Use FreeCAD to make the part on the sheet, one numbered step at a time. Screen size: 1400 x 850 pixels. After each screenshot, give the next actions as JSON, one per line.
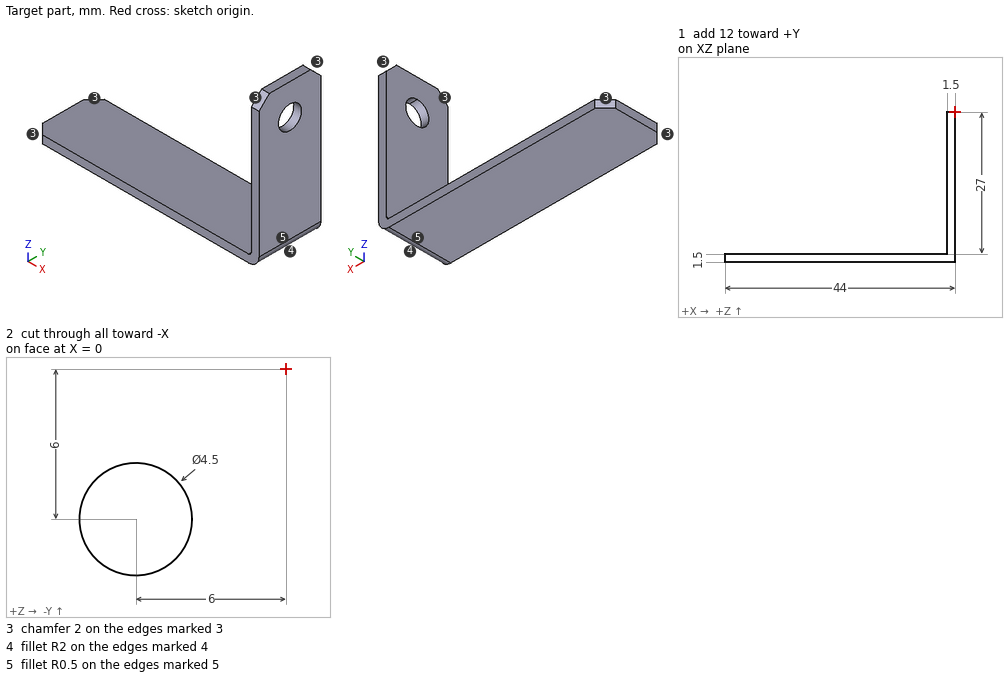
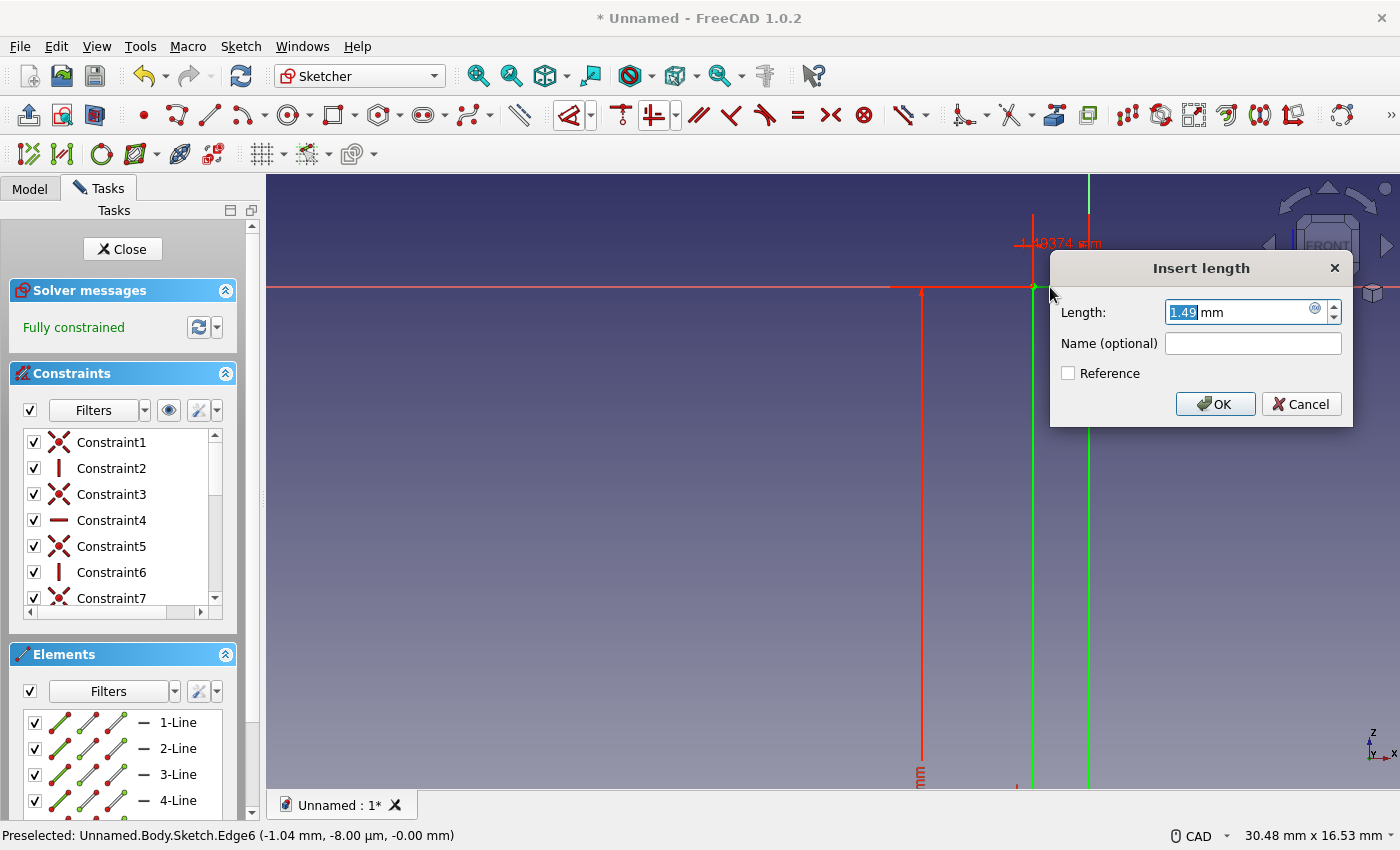
{"action": "type", "text": "1.5"}
{"action": "key", "text": "Return"}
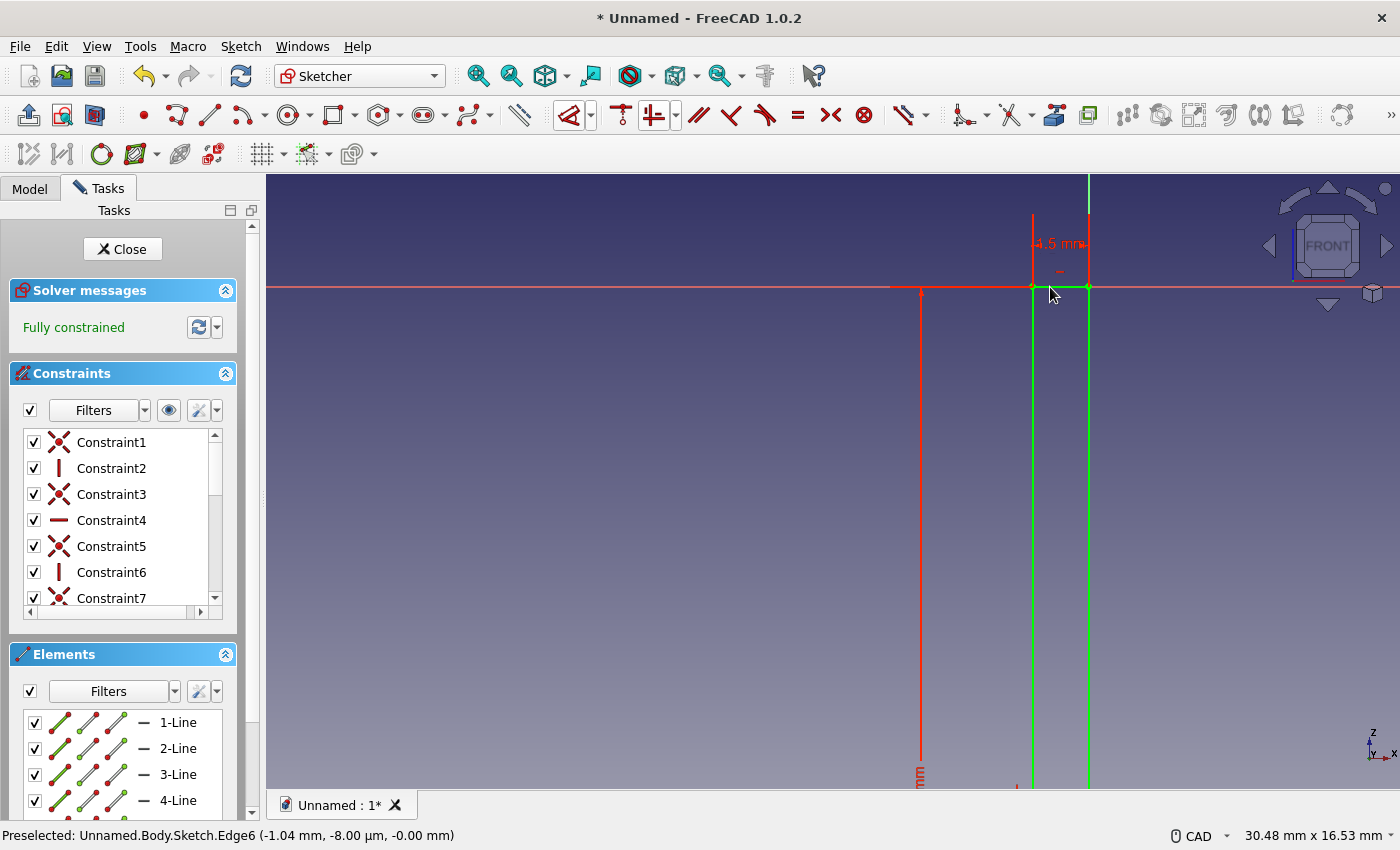
{"action": "left_click", "coordinate": [123, 249]}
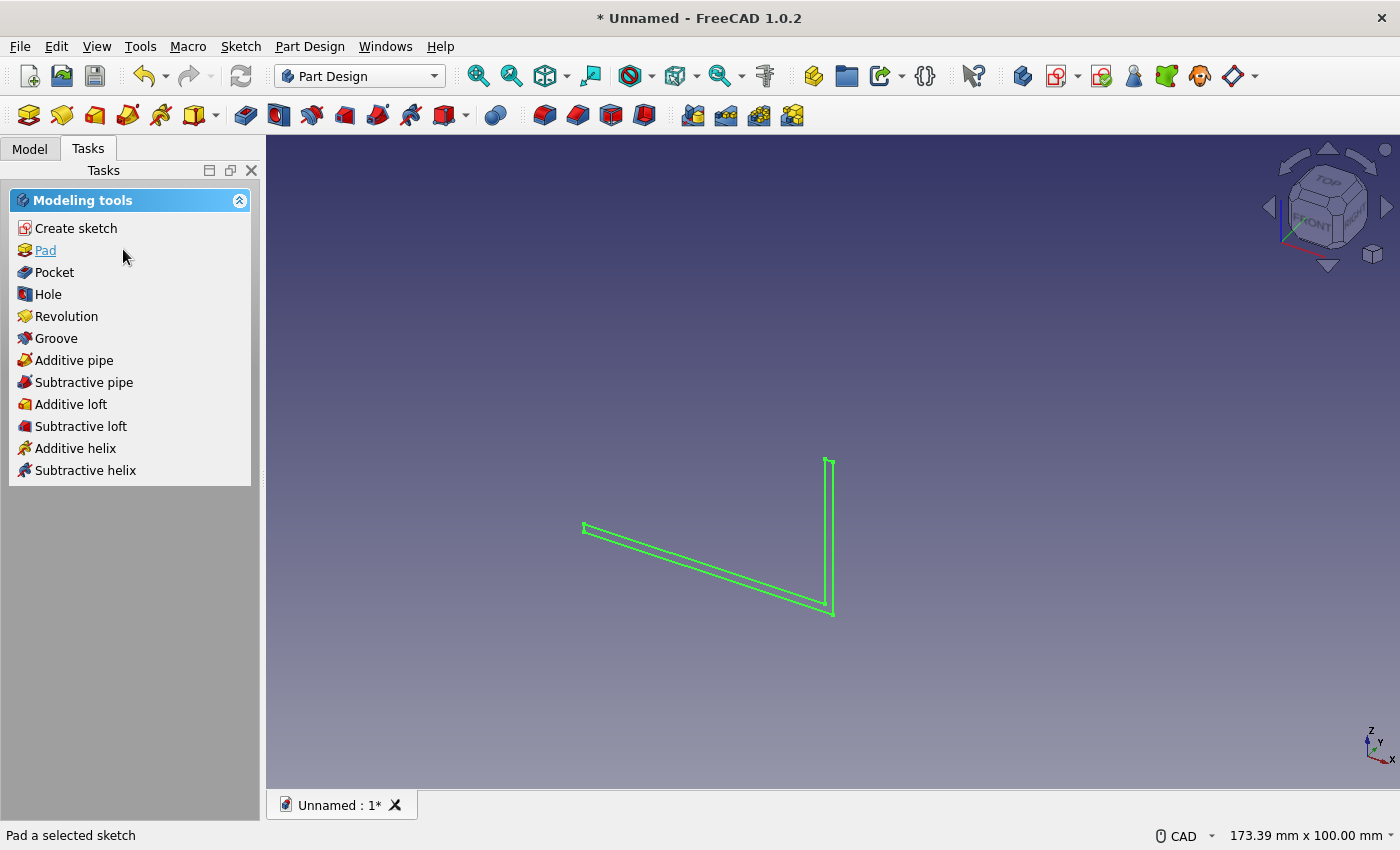
{"action": "left_click", "coordinate": [29, 116]}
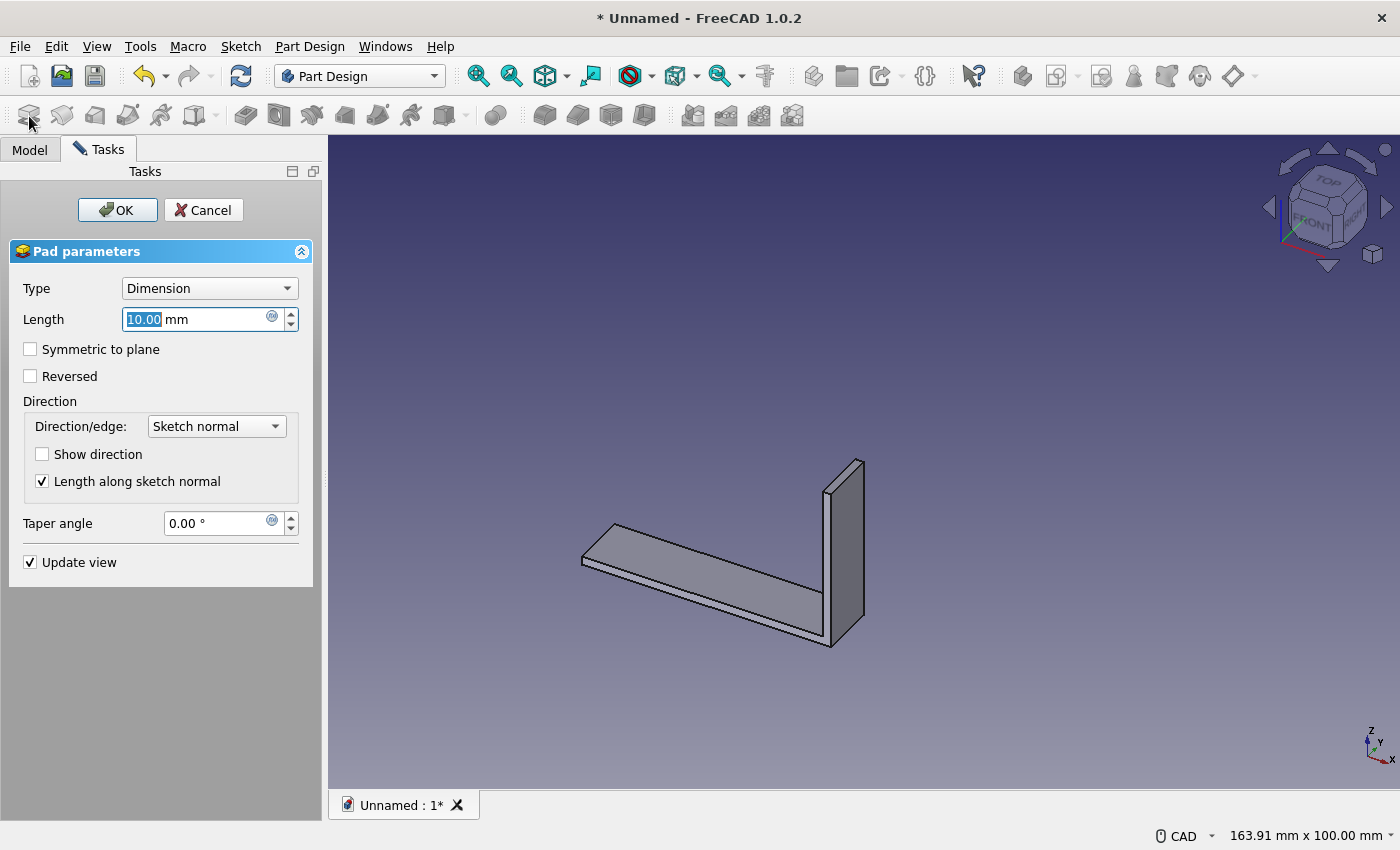
{"action": "type", "text": "12"}
{"action": "key", "text": "Tab"}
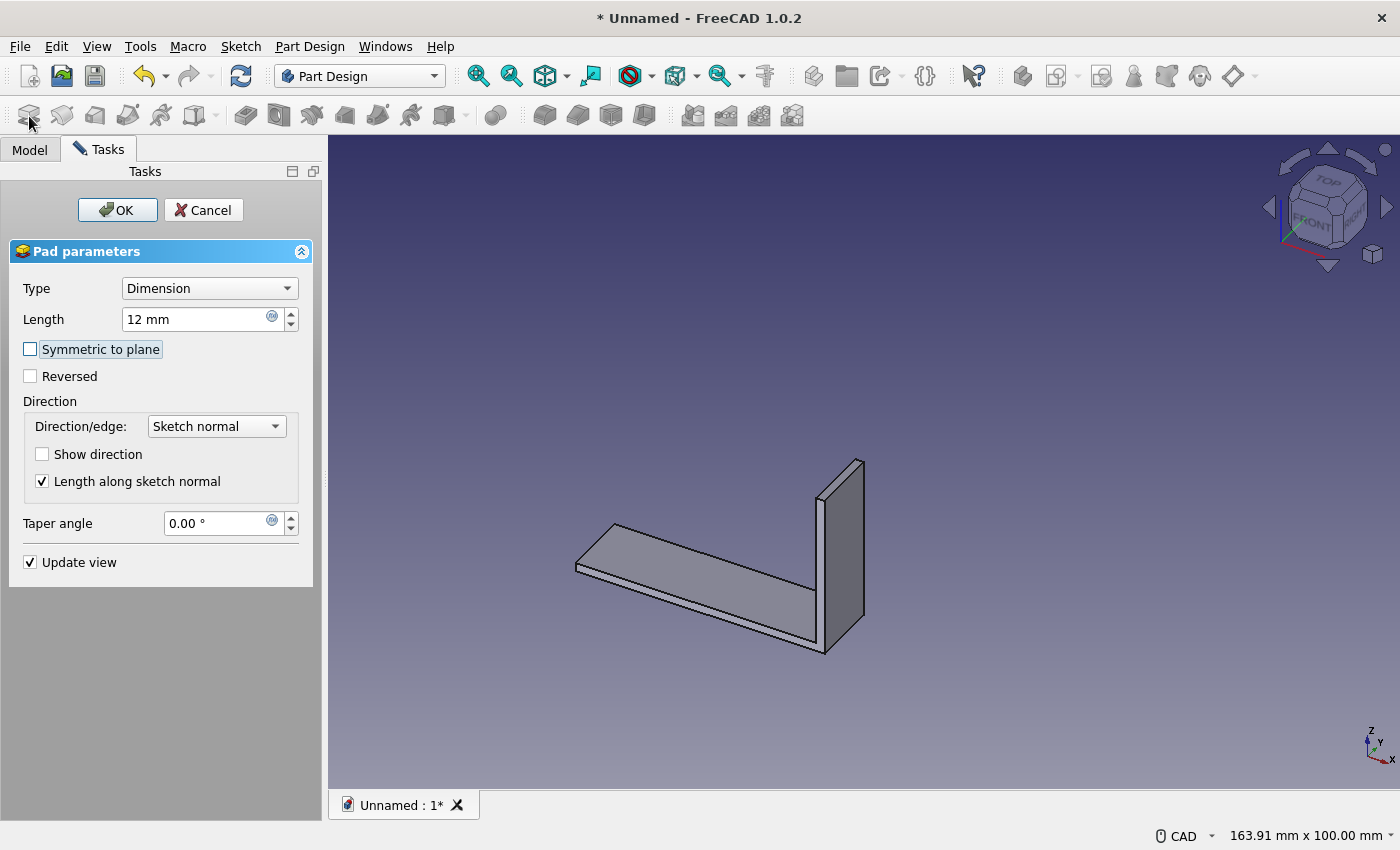
{"action": "left_click", "coordinate": [31, 376]}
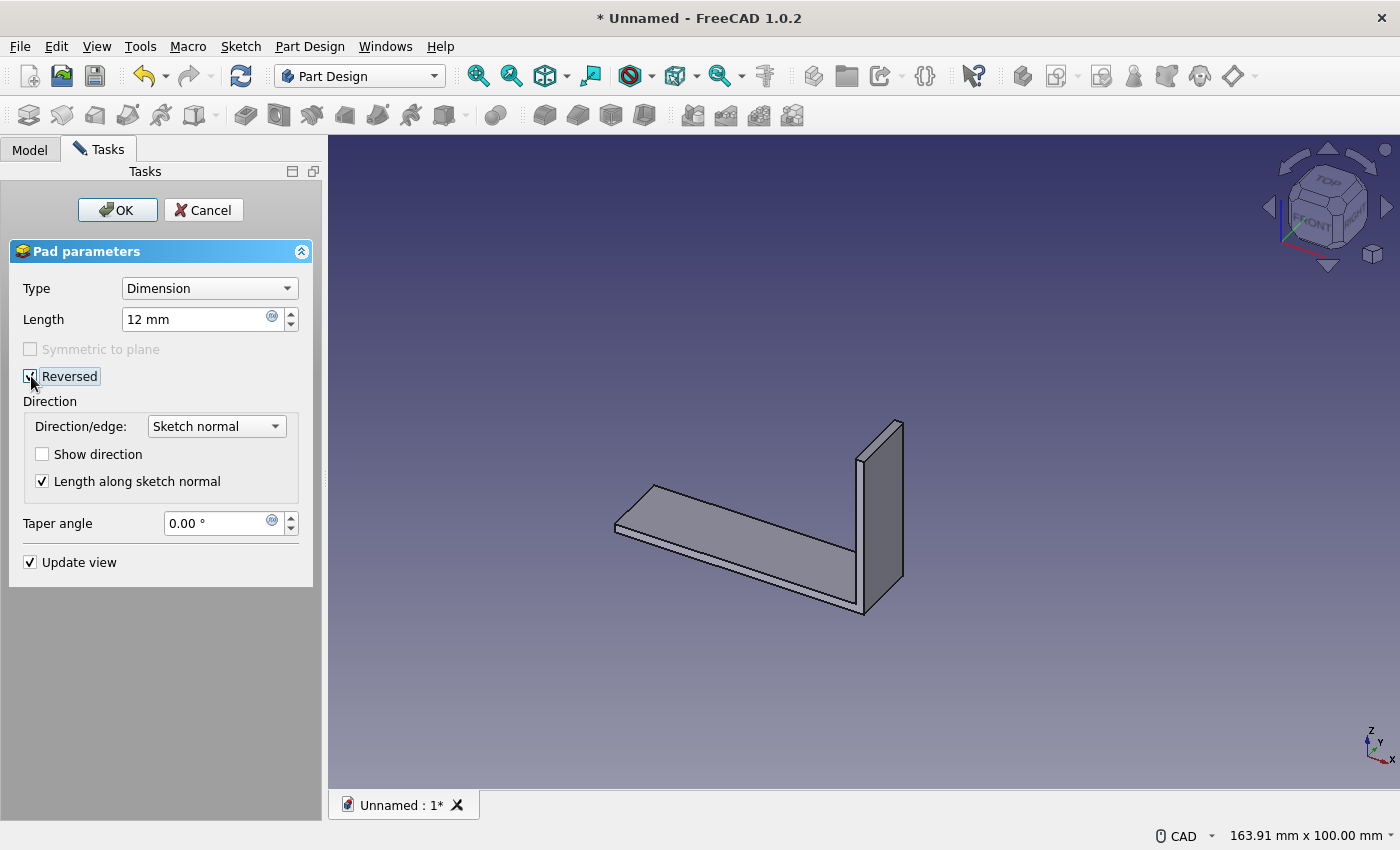
{"action": "left_click", "coordinate": [118, 210]}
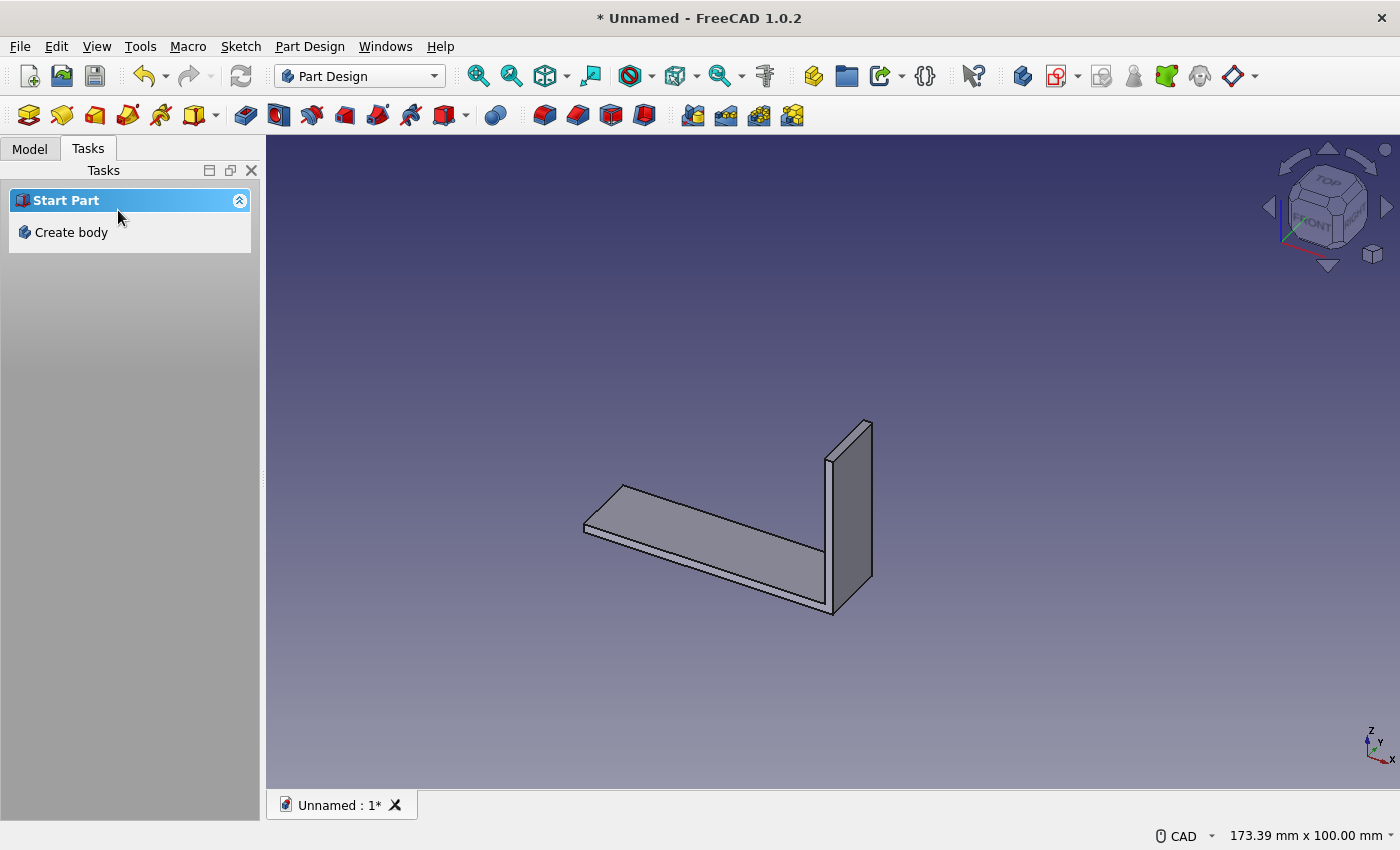
{"action": "left_click", "coordinate": [479, 76]}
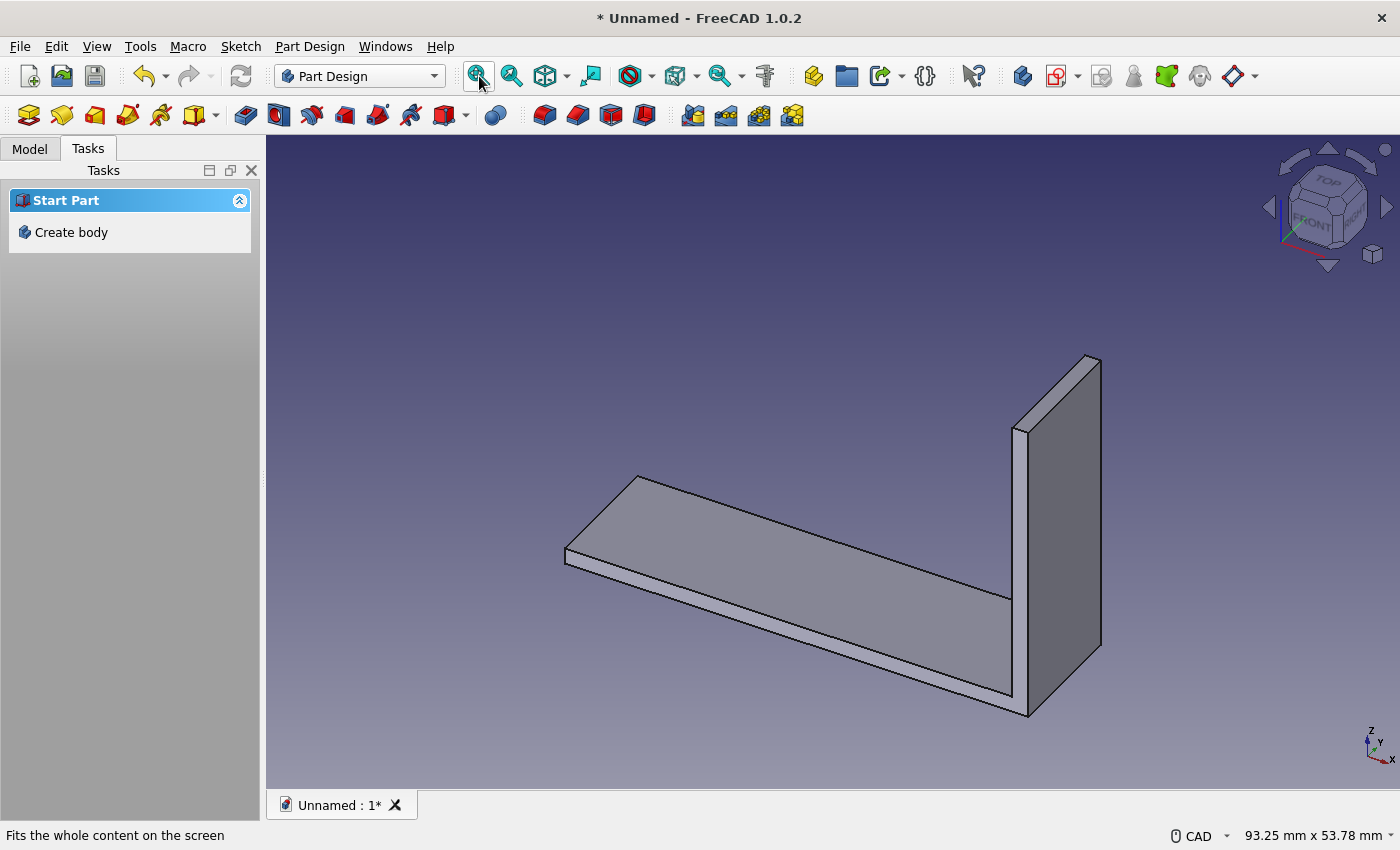
{"action": "left_click", "coordinate": [1065, 457]}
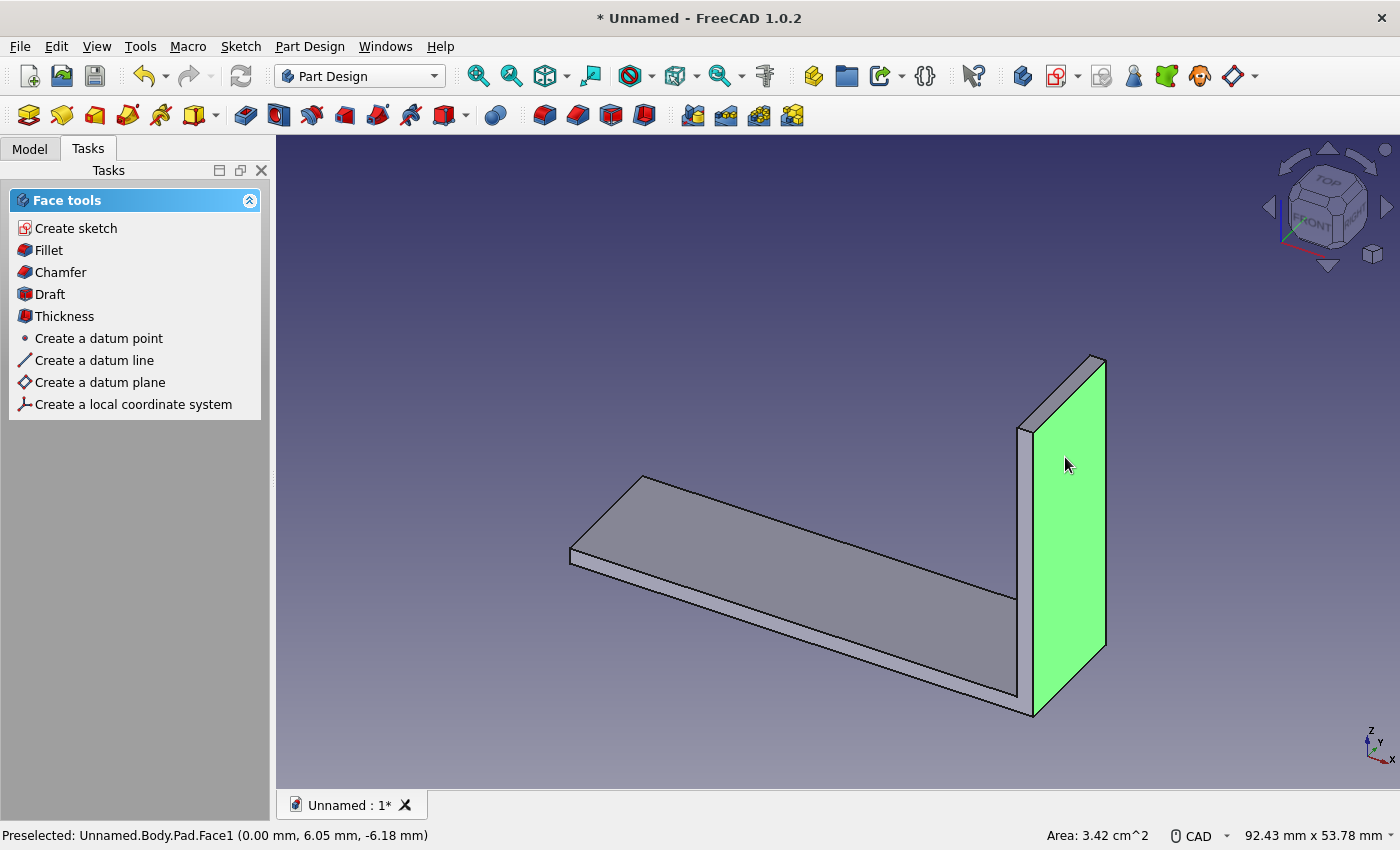
{"action": "left_click", "coordinate": [1056, 76]}